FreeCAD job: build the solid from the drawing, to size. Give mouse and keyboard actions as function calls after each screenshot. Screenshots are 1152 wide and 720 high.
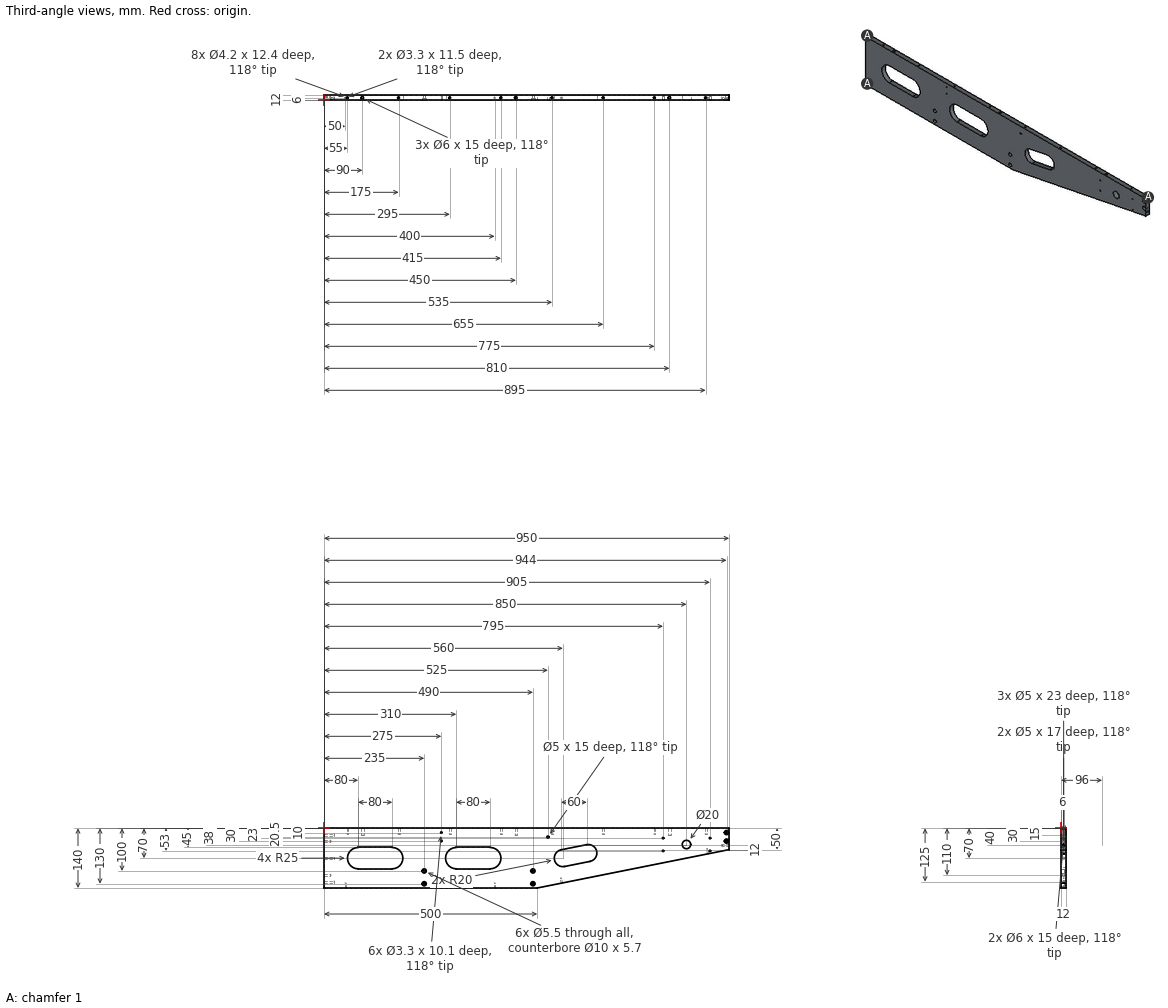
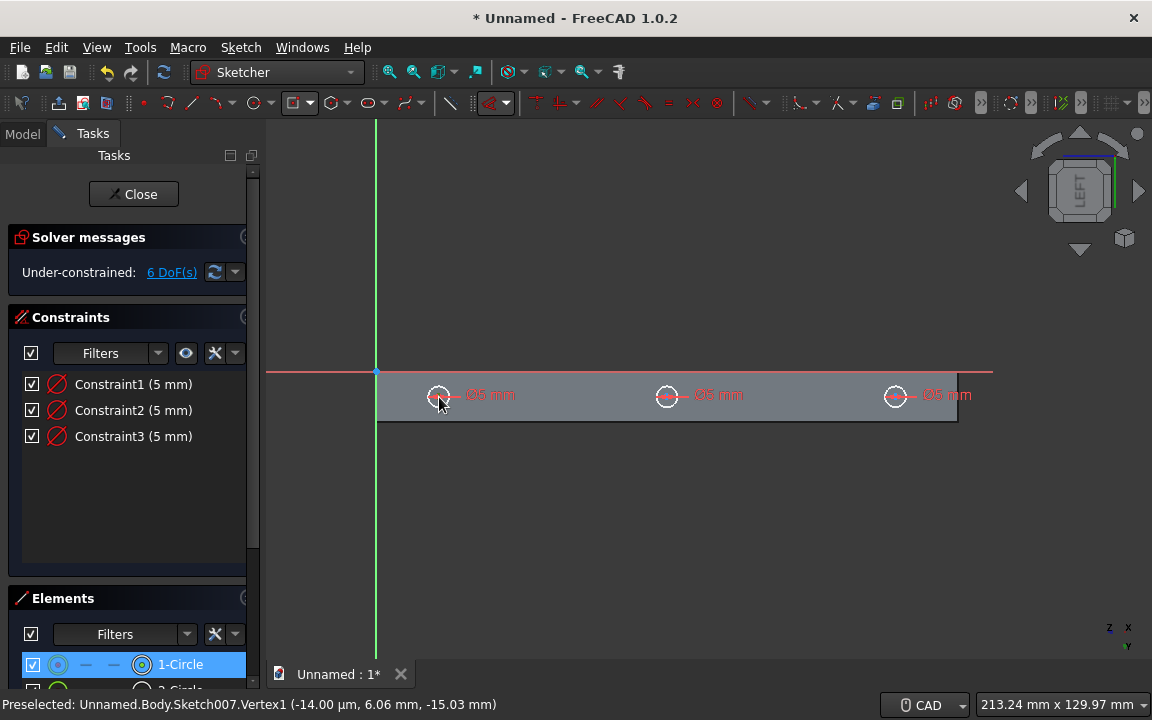
click(667, 397)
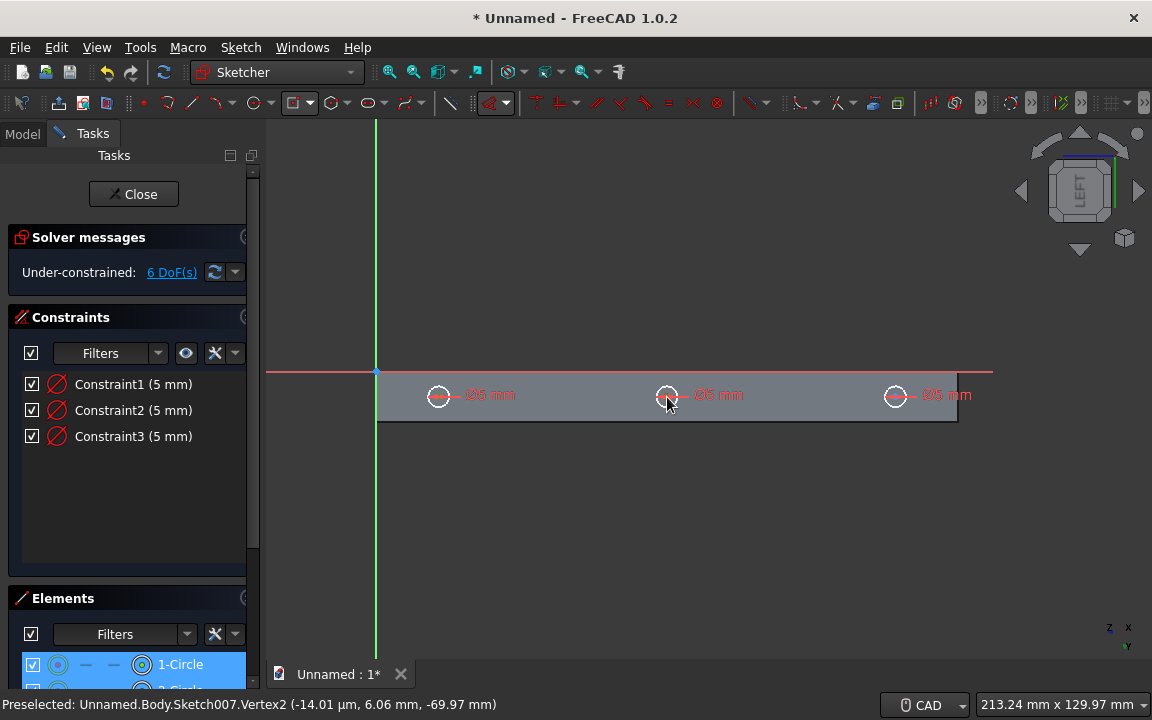
key(h)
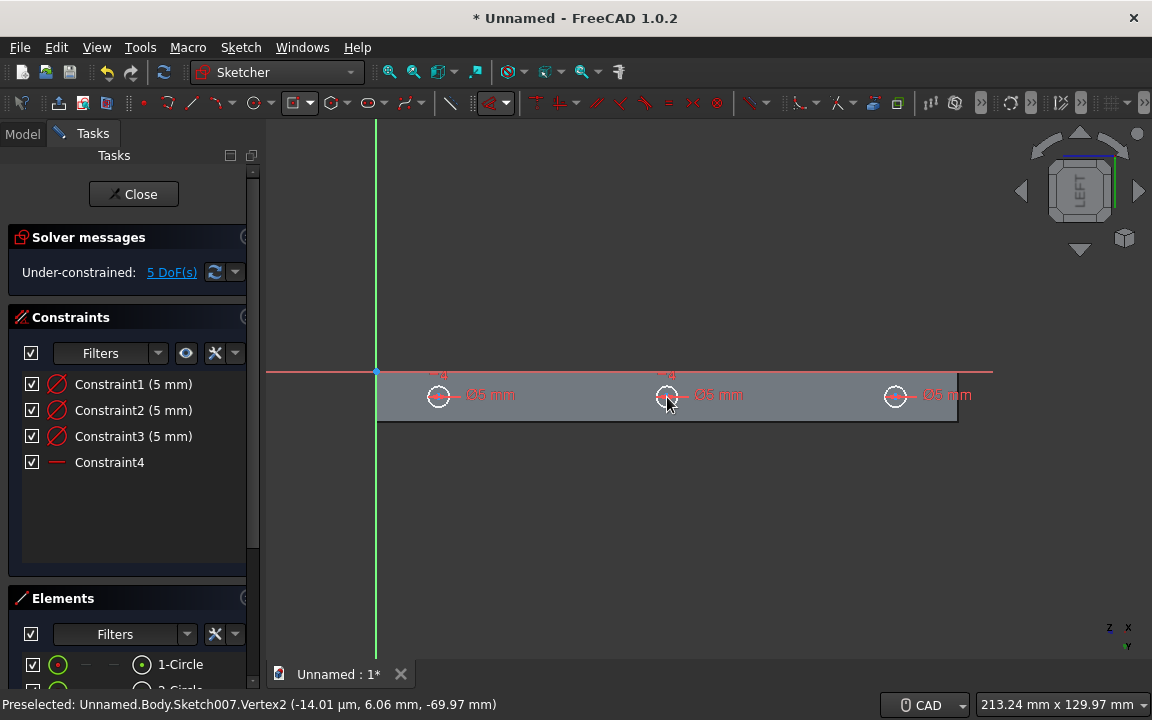
click(667, 397)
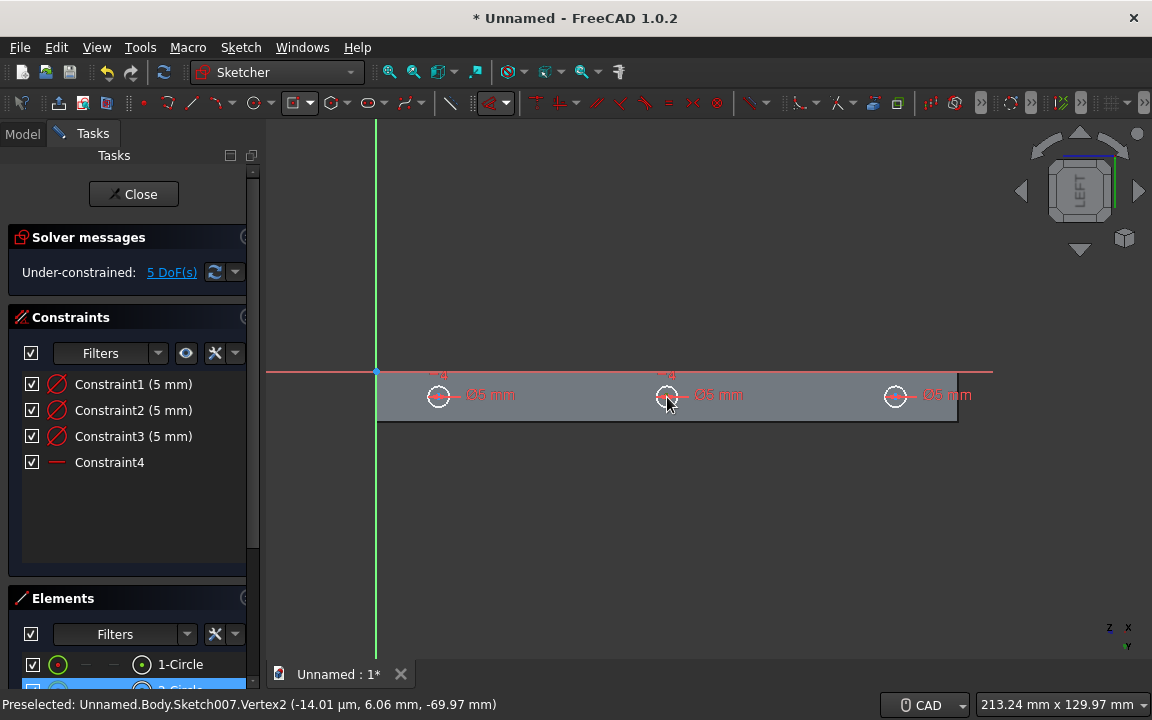
click(895, 397)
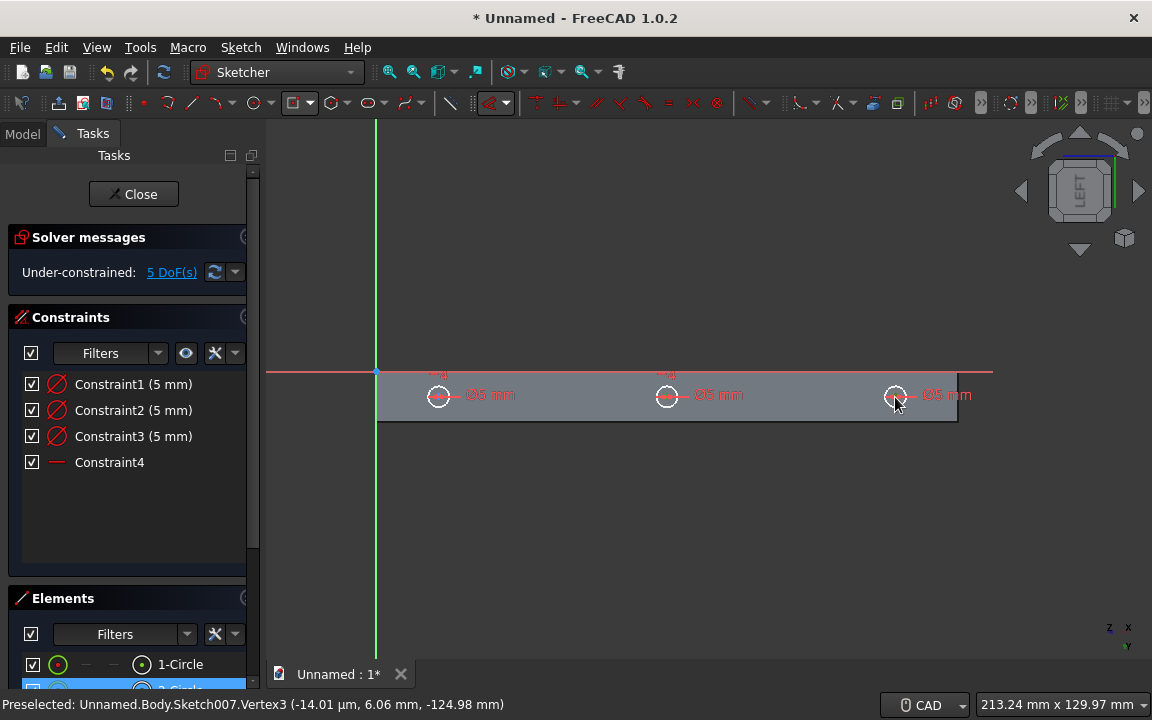
key(h)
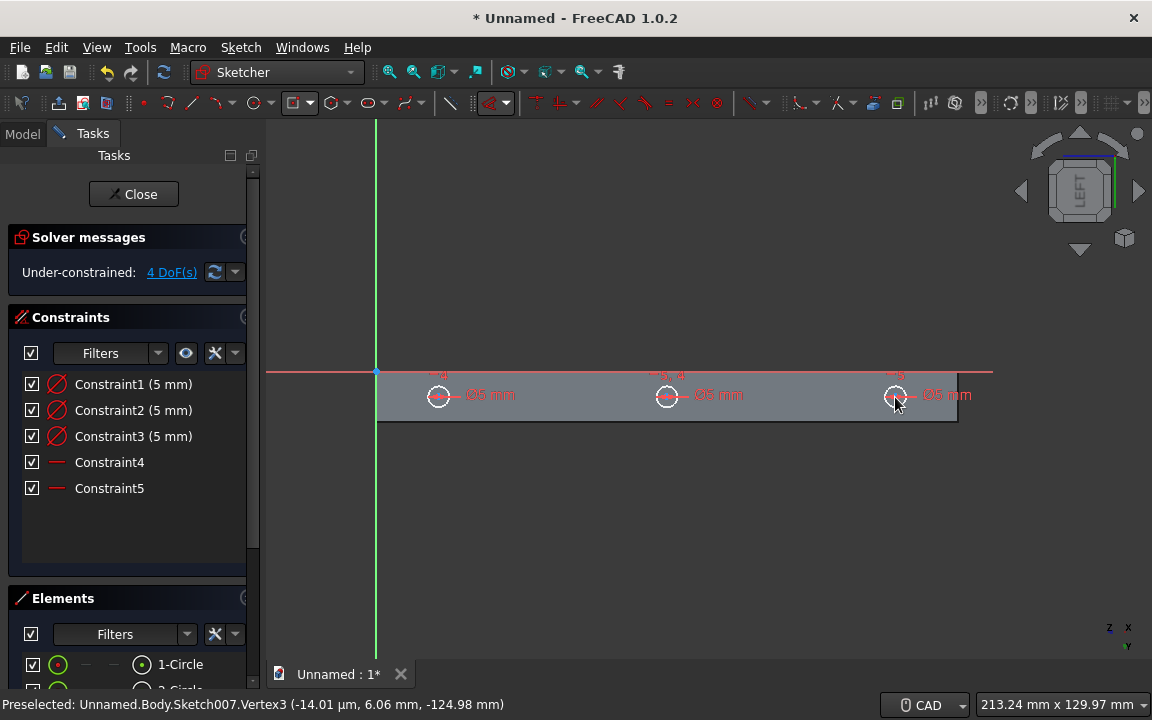
scroll(439, 397, up, 3)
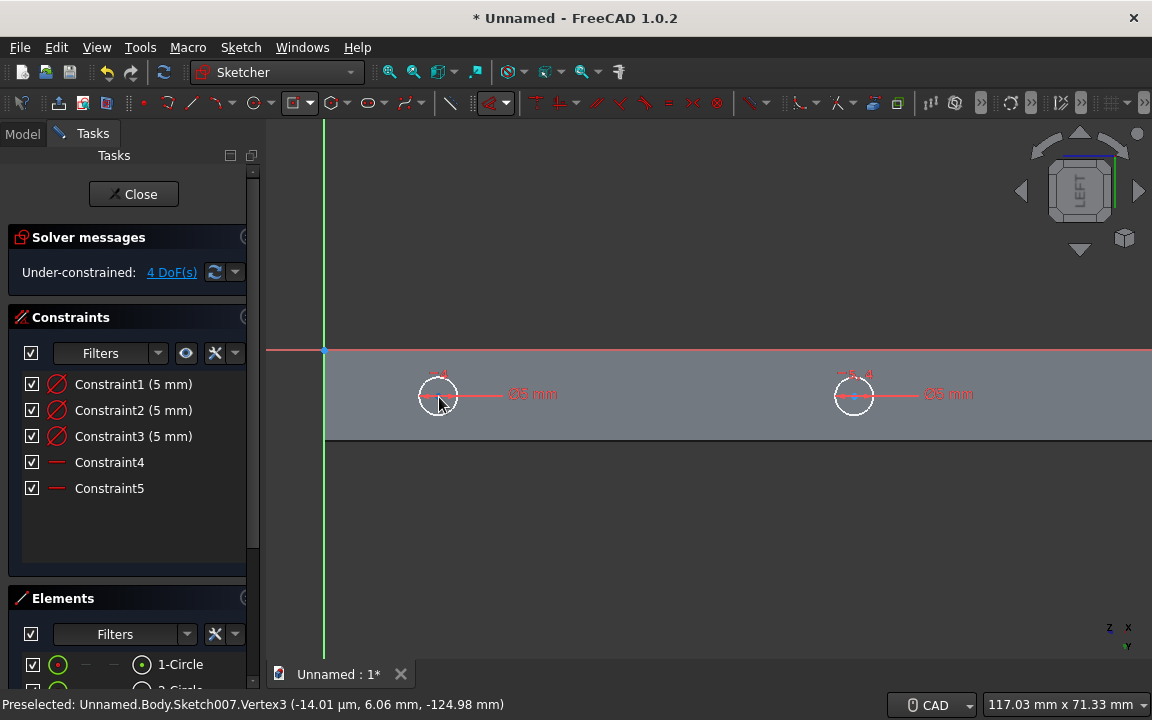
click(438, 396)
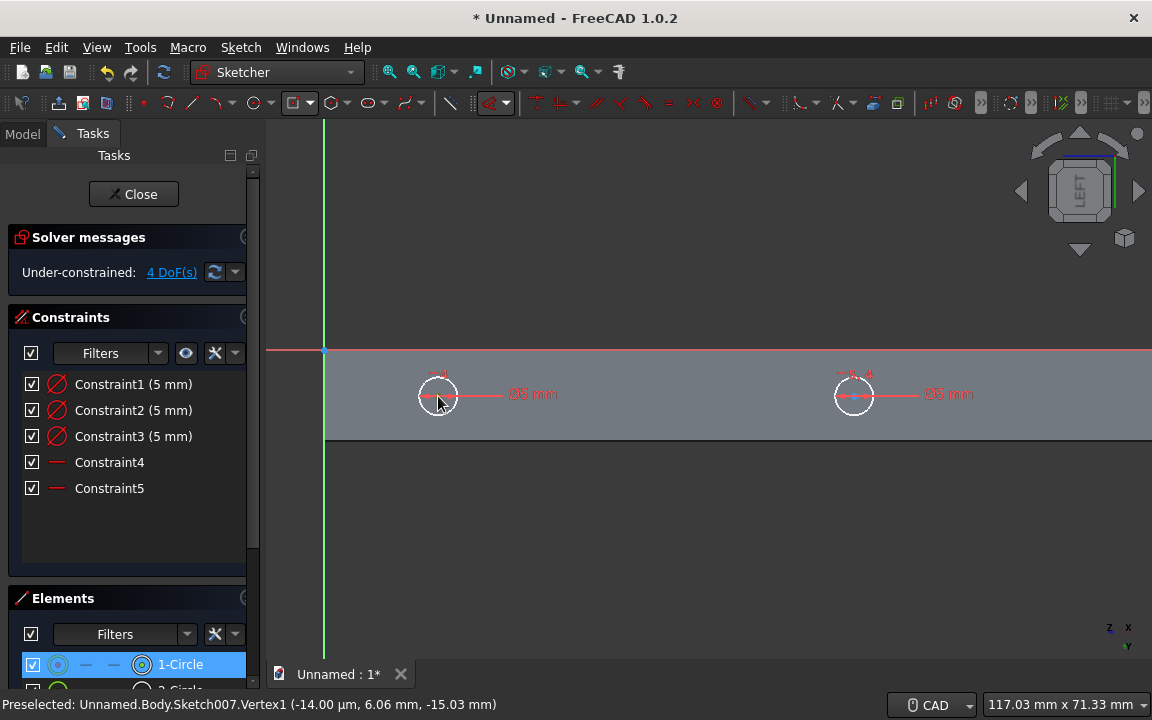
key(i)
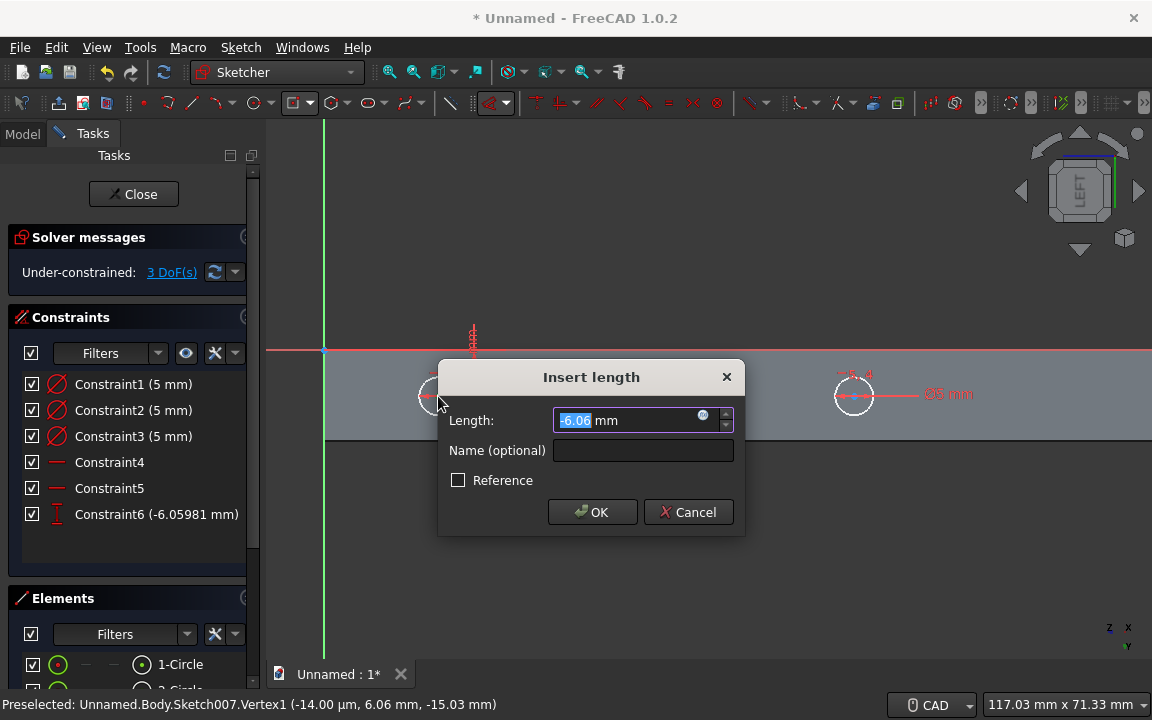
text(-6)
key(Return)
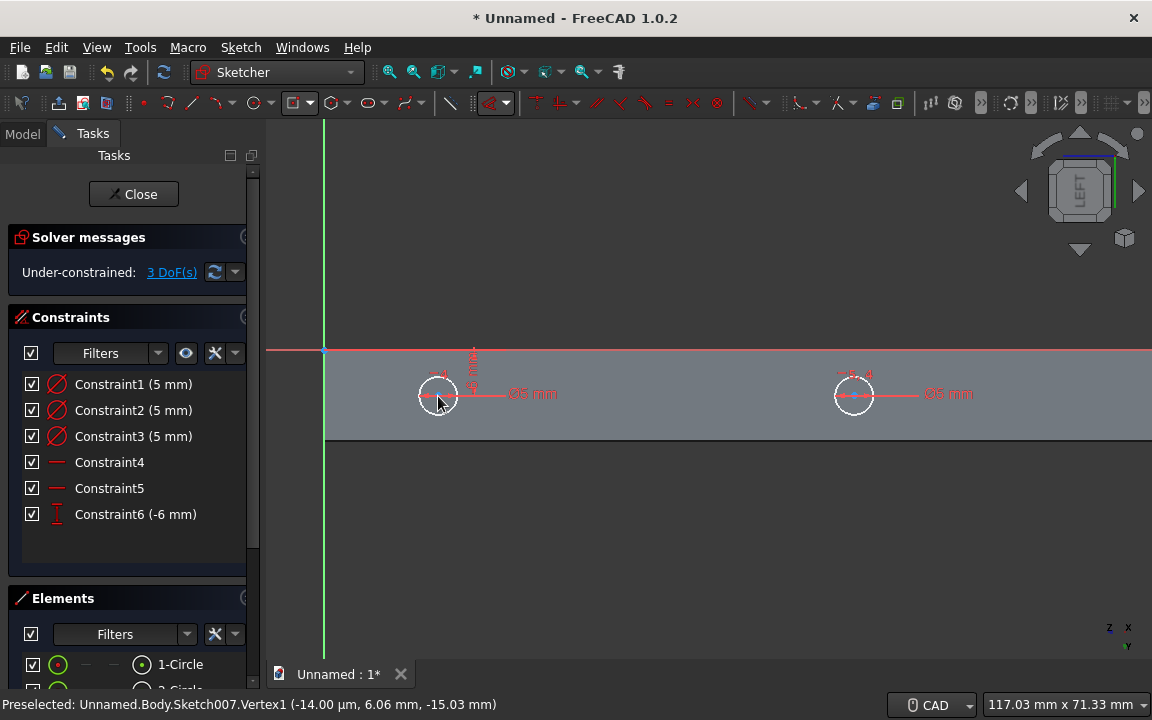
click(438, 396)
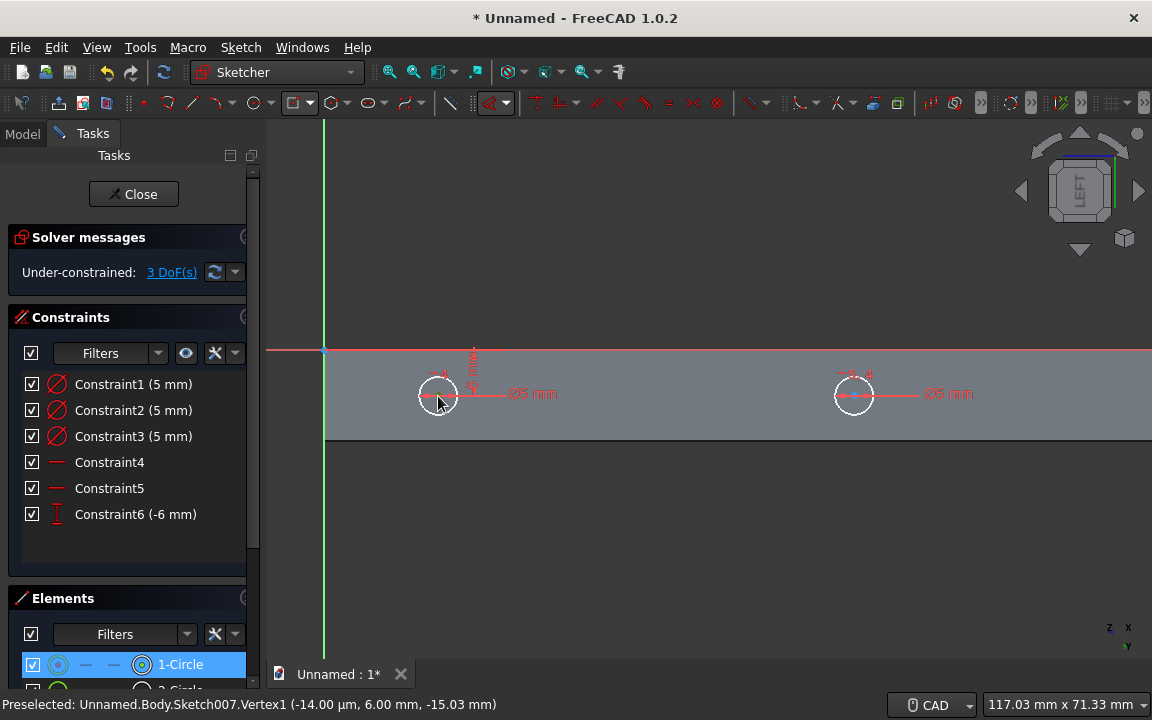
key(l)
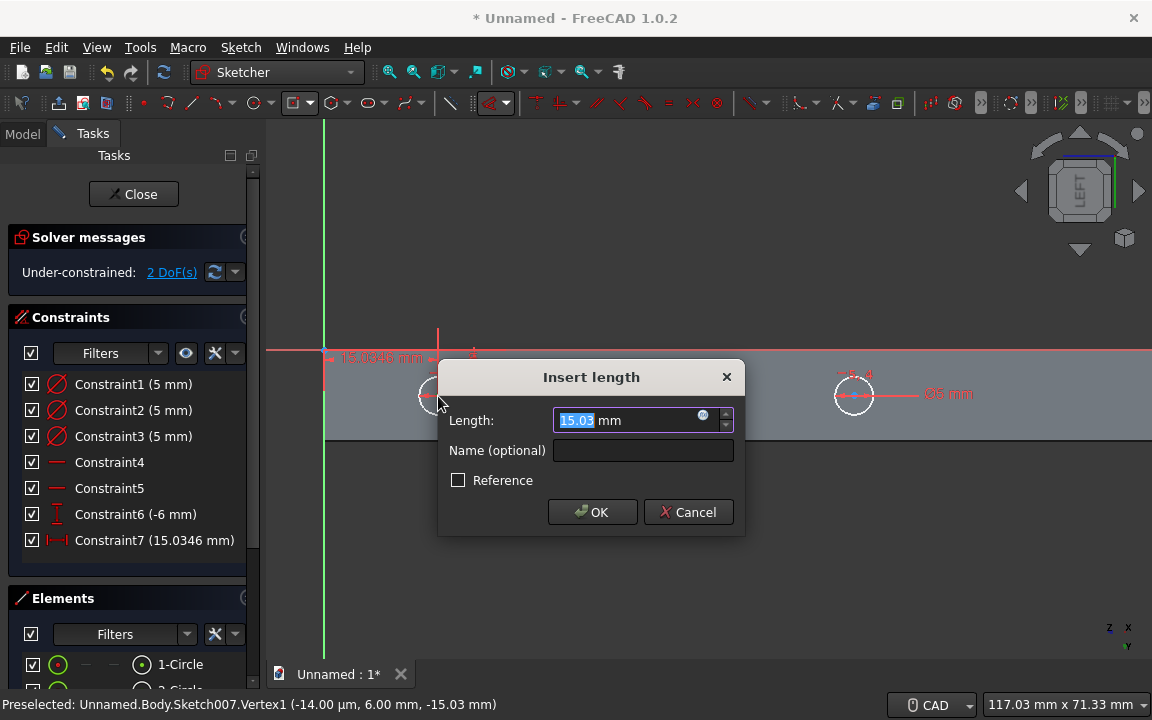
text(15)
key(Return)